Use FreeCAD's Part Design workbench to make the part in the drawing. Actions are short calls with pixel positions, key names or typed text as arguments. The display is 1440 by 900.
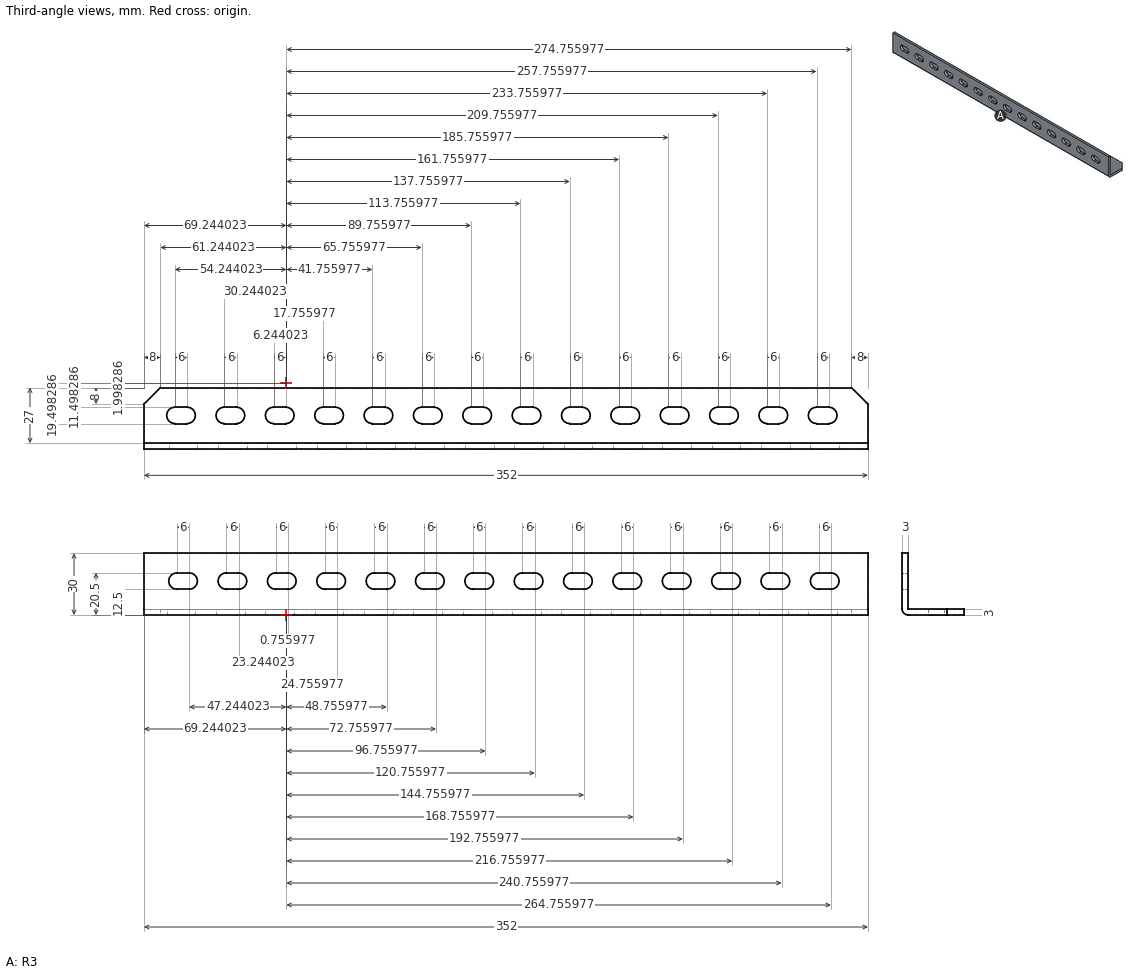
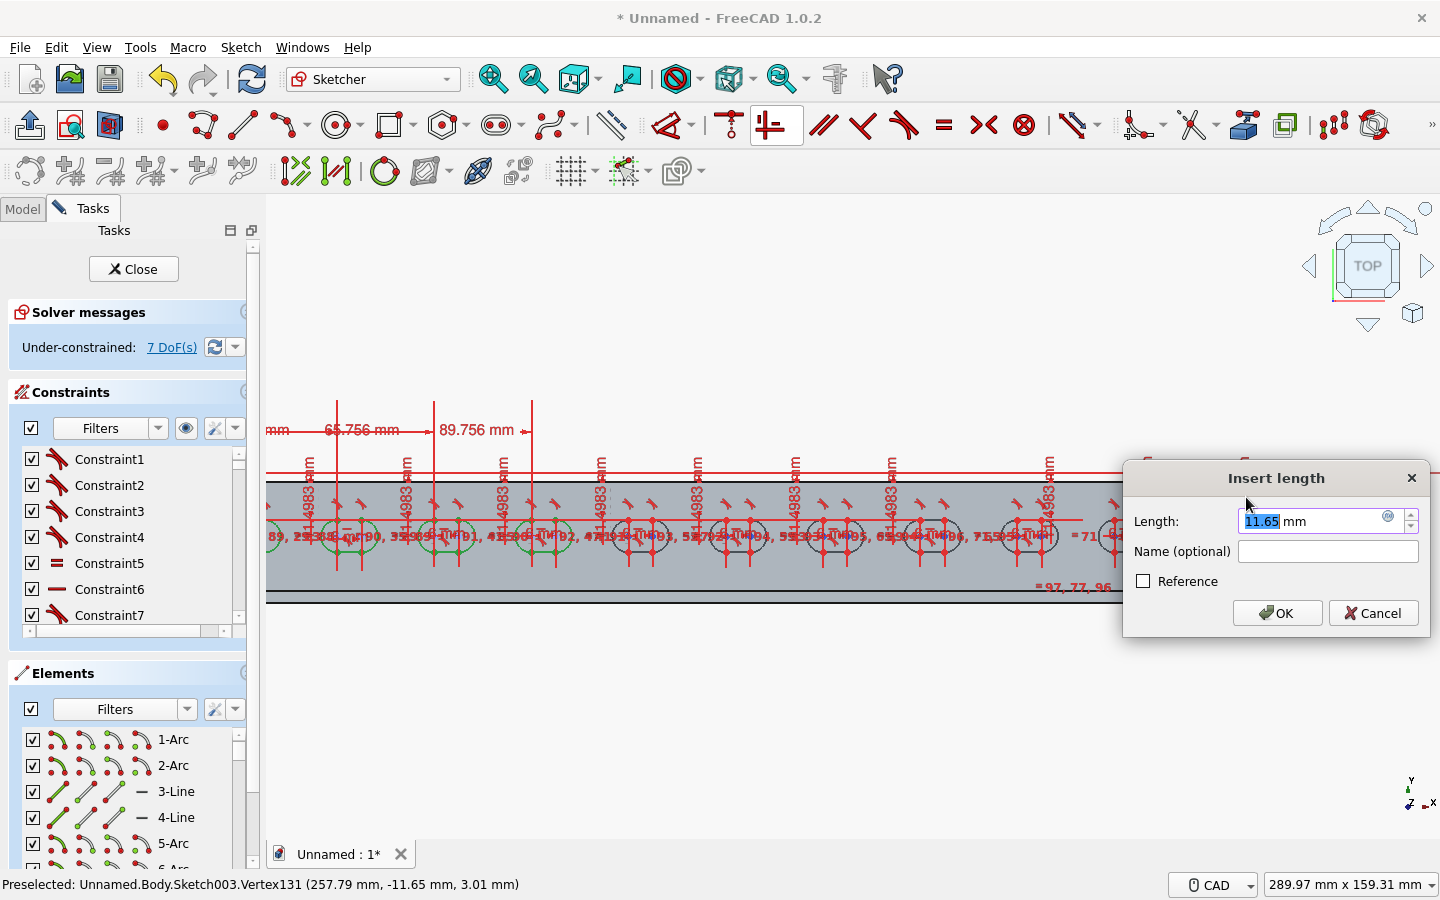
text(11.498286)
key(Return)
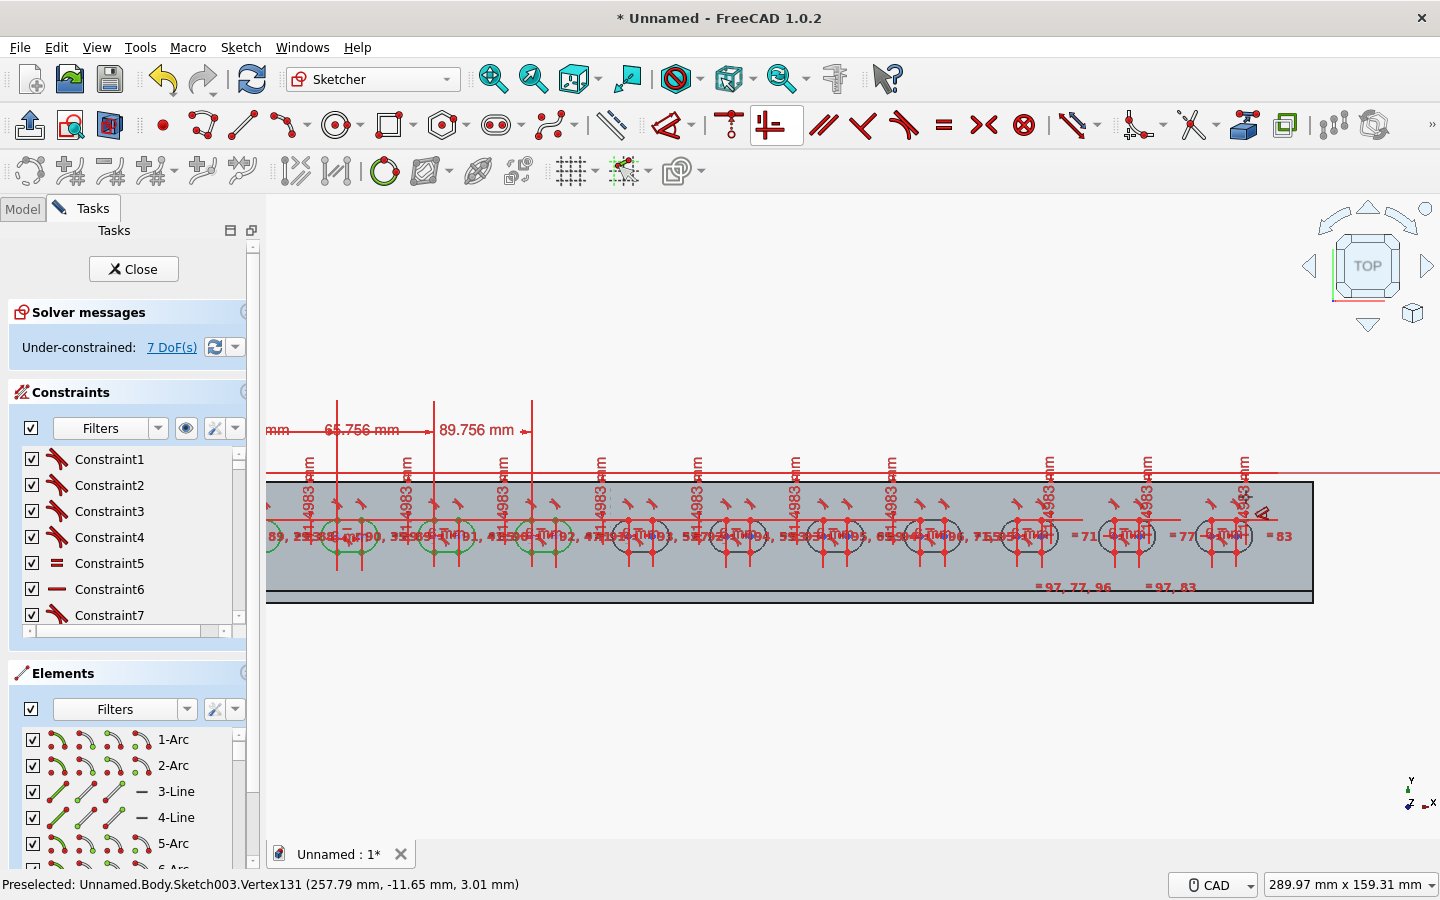
click(629, 520)
click(578, 439)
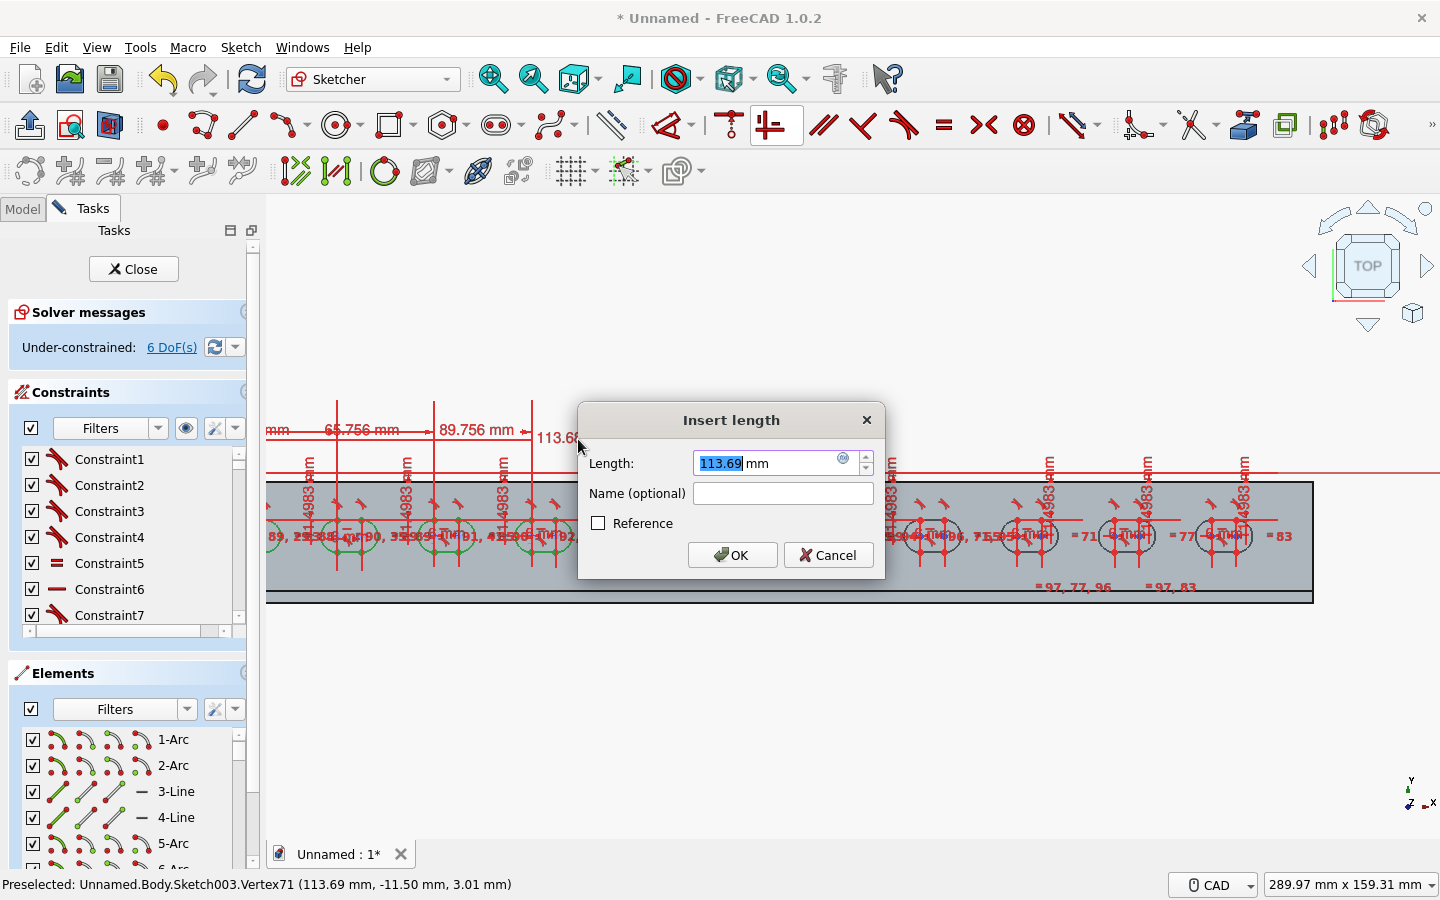
text(113.755977)
key(Return)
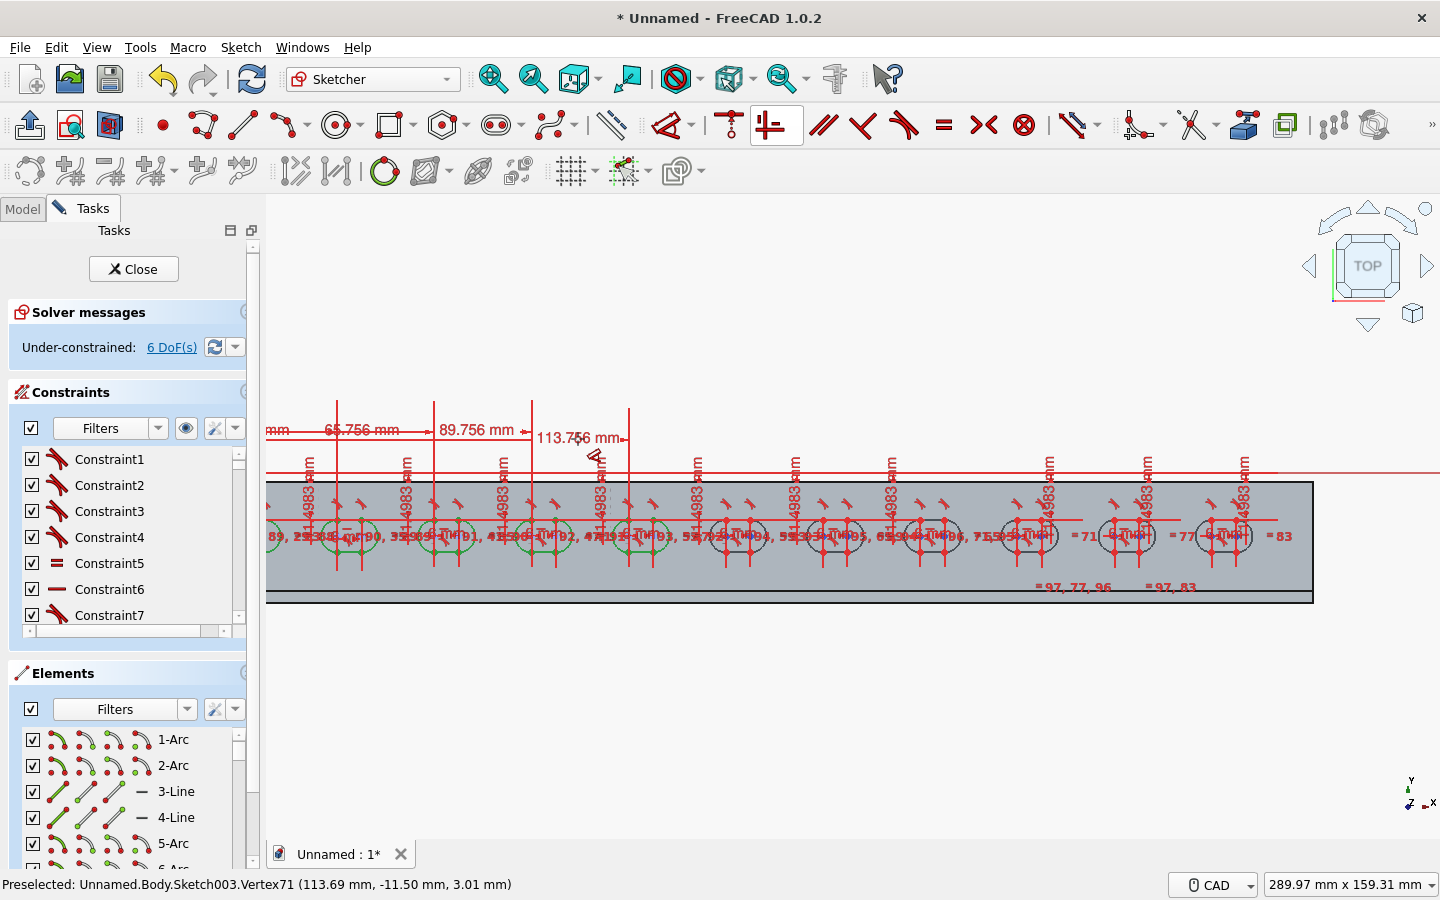
click(726, 520)
click(661, 439)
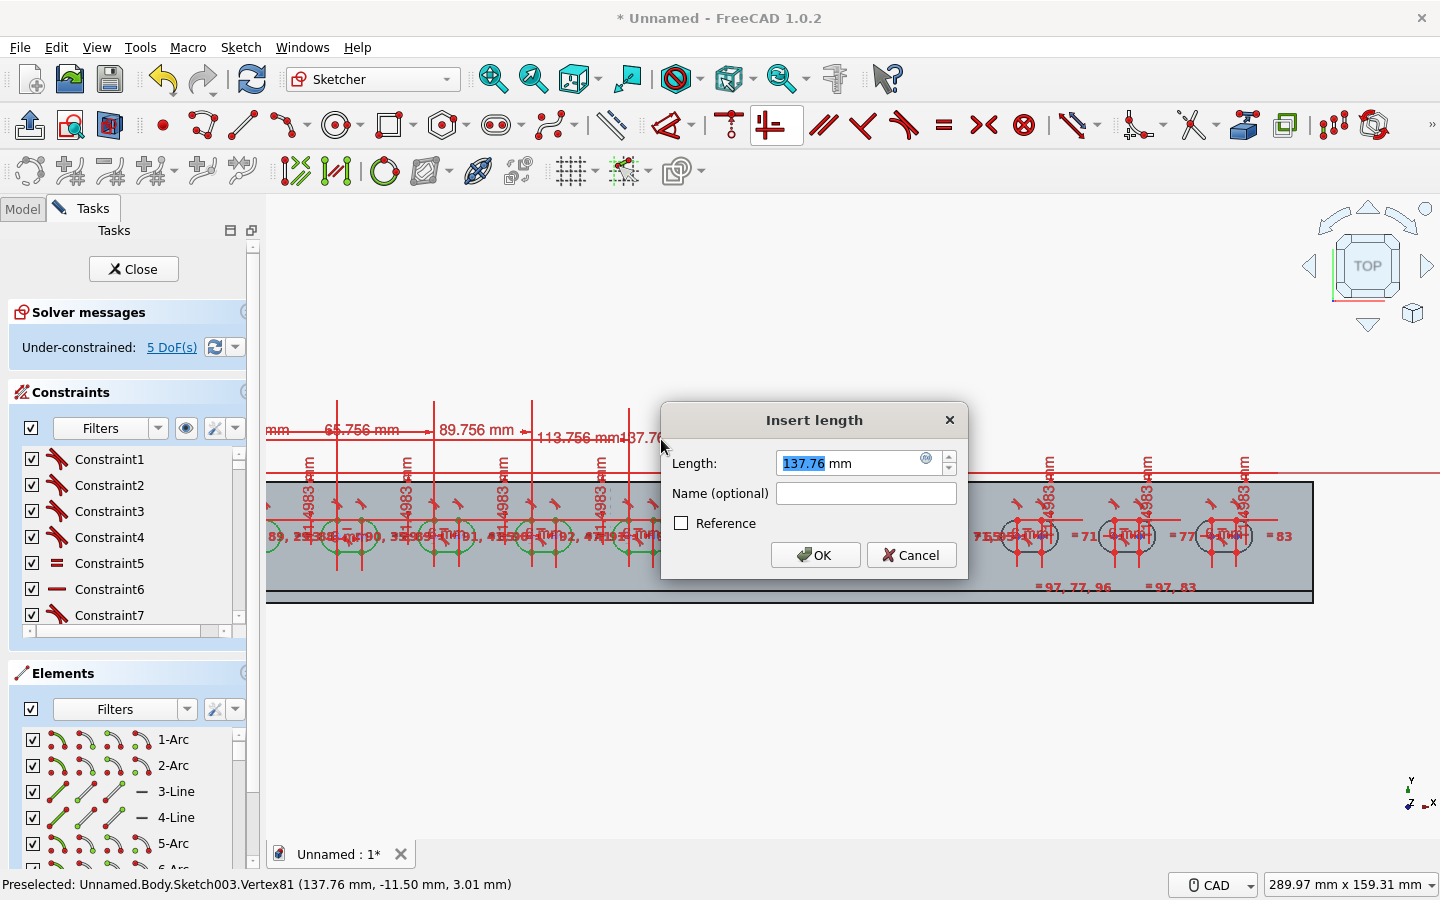
text(137.755977)
key(Return)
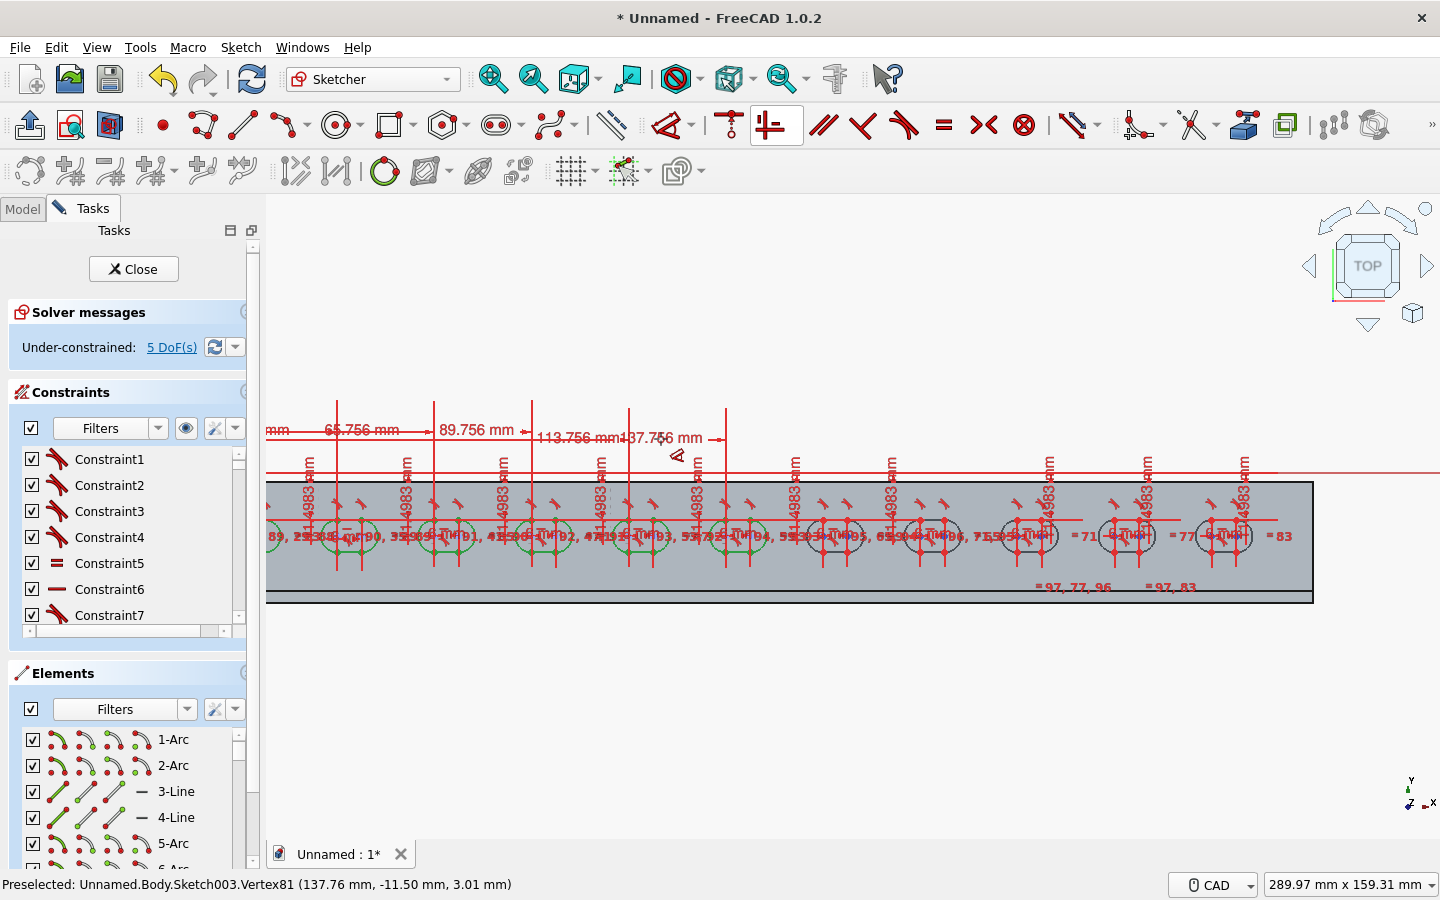
click(823, 520)
click(744, 439)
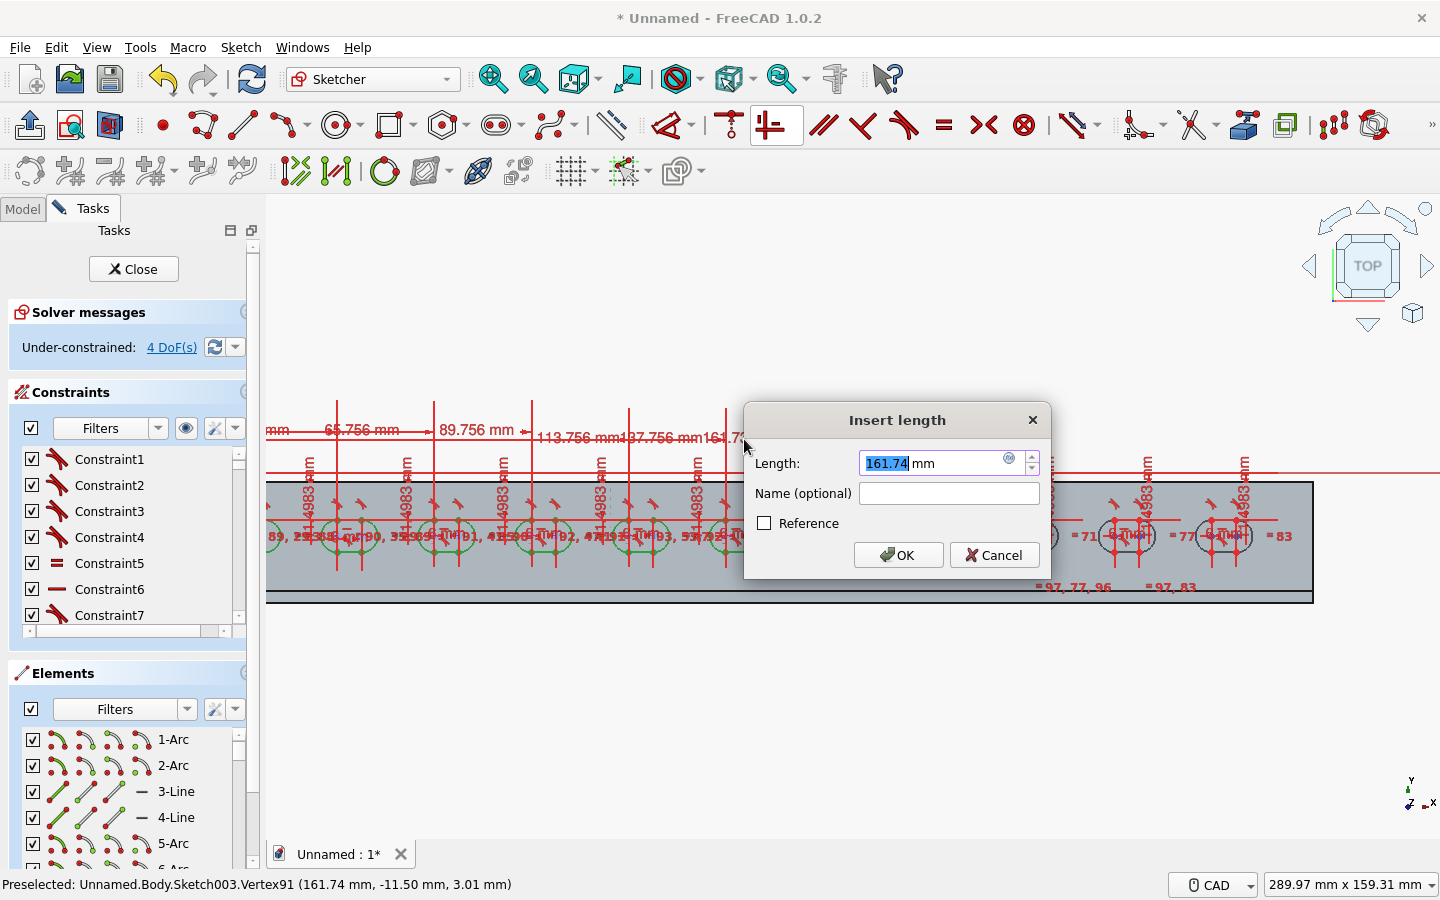
text(161.755977)
key(Return)